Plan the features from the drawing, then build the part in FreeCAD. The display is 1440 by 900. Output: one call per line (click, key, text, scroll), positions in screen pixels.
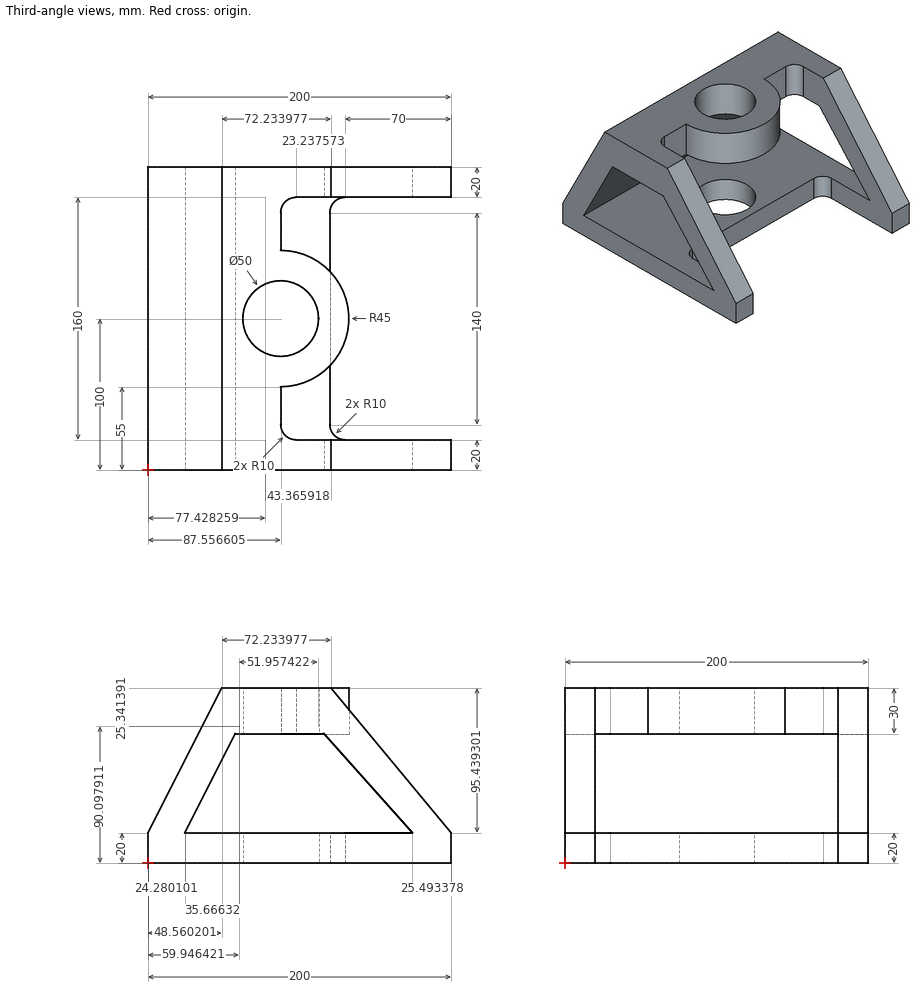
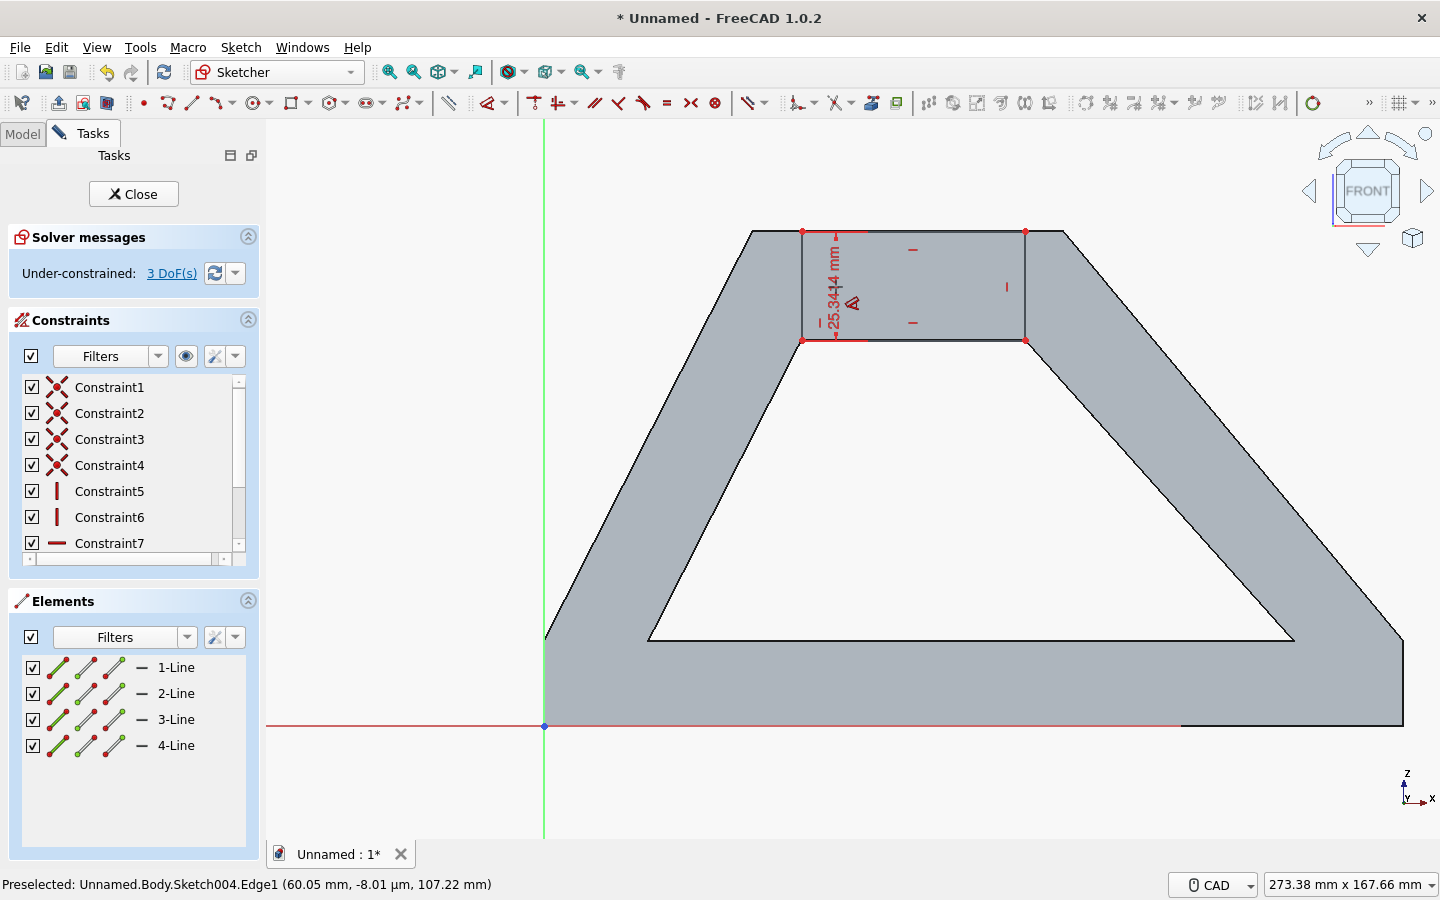
click(869, 341)
click(913, 307)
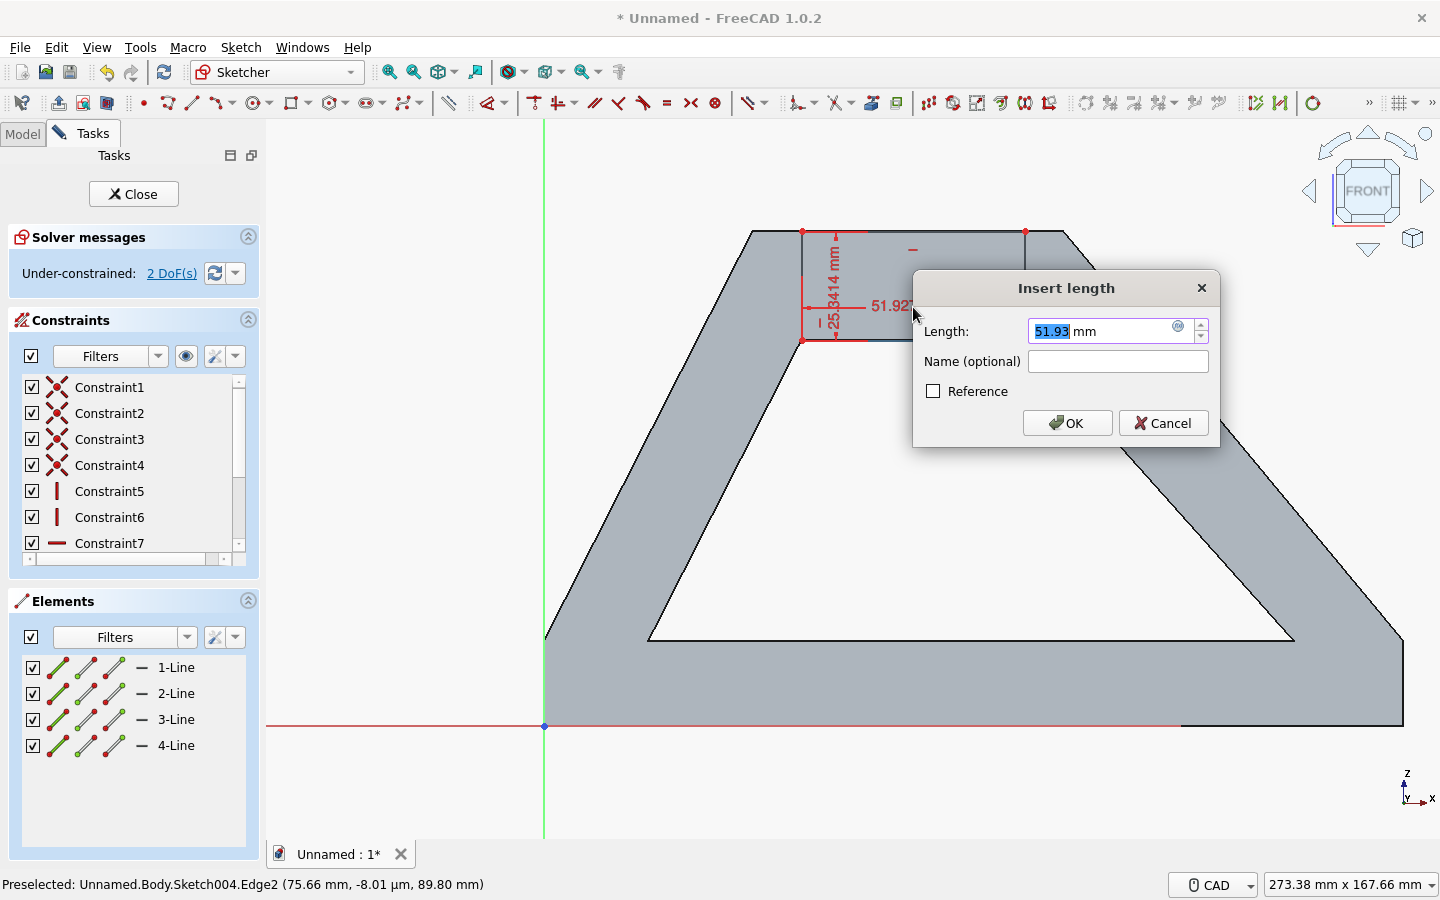
text(51.957422)
key(Return)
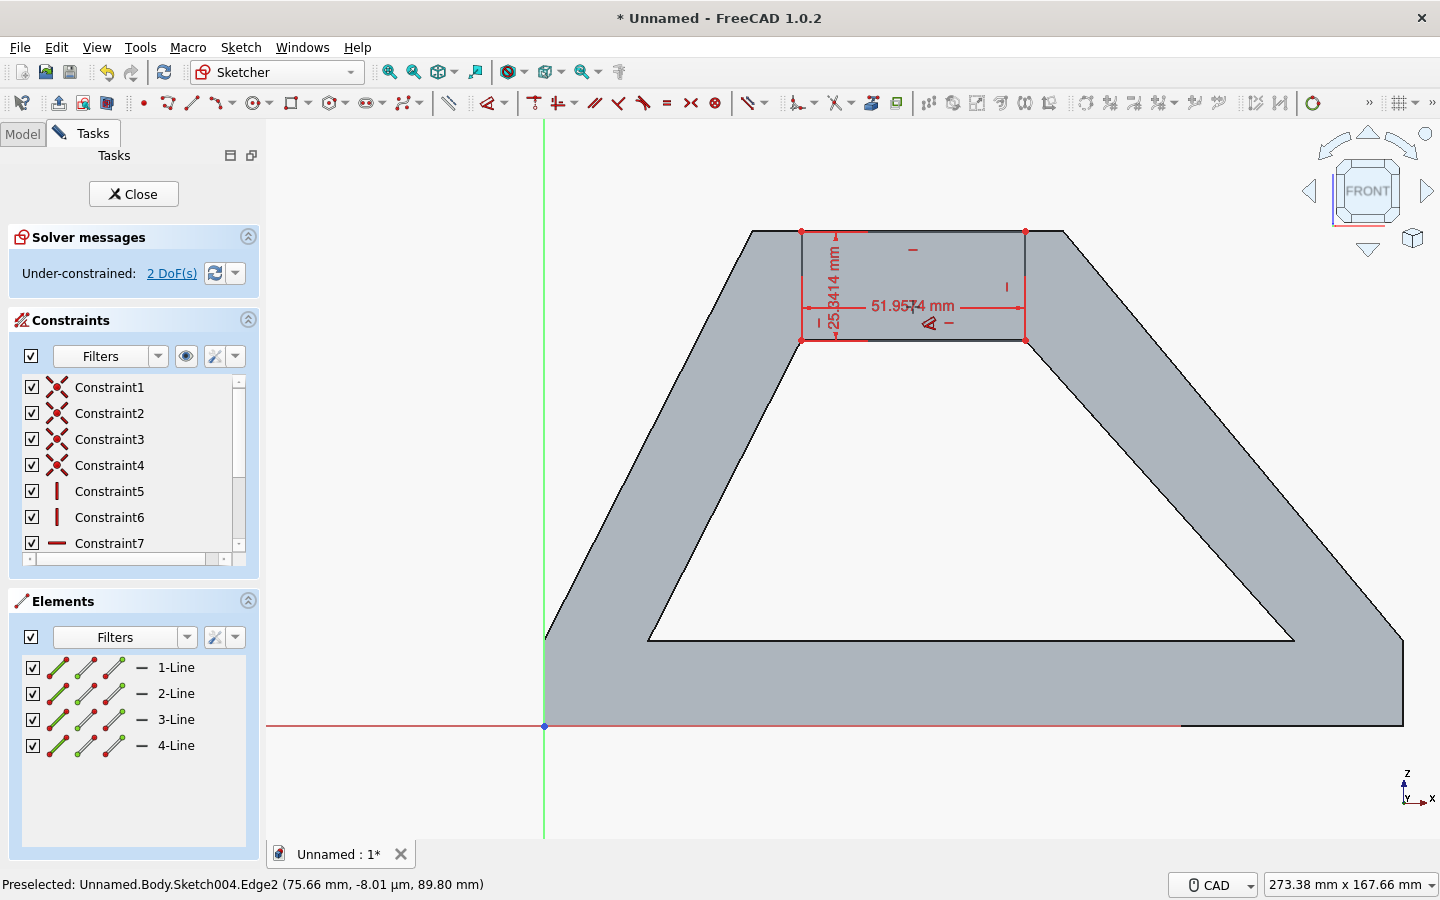
click(802, 232)
click(673, 760)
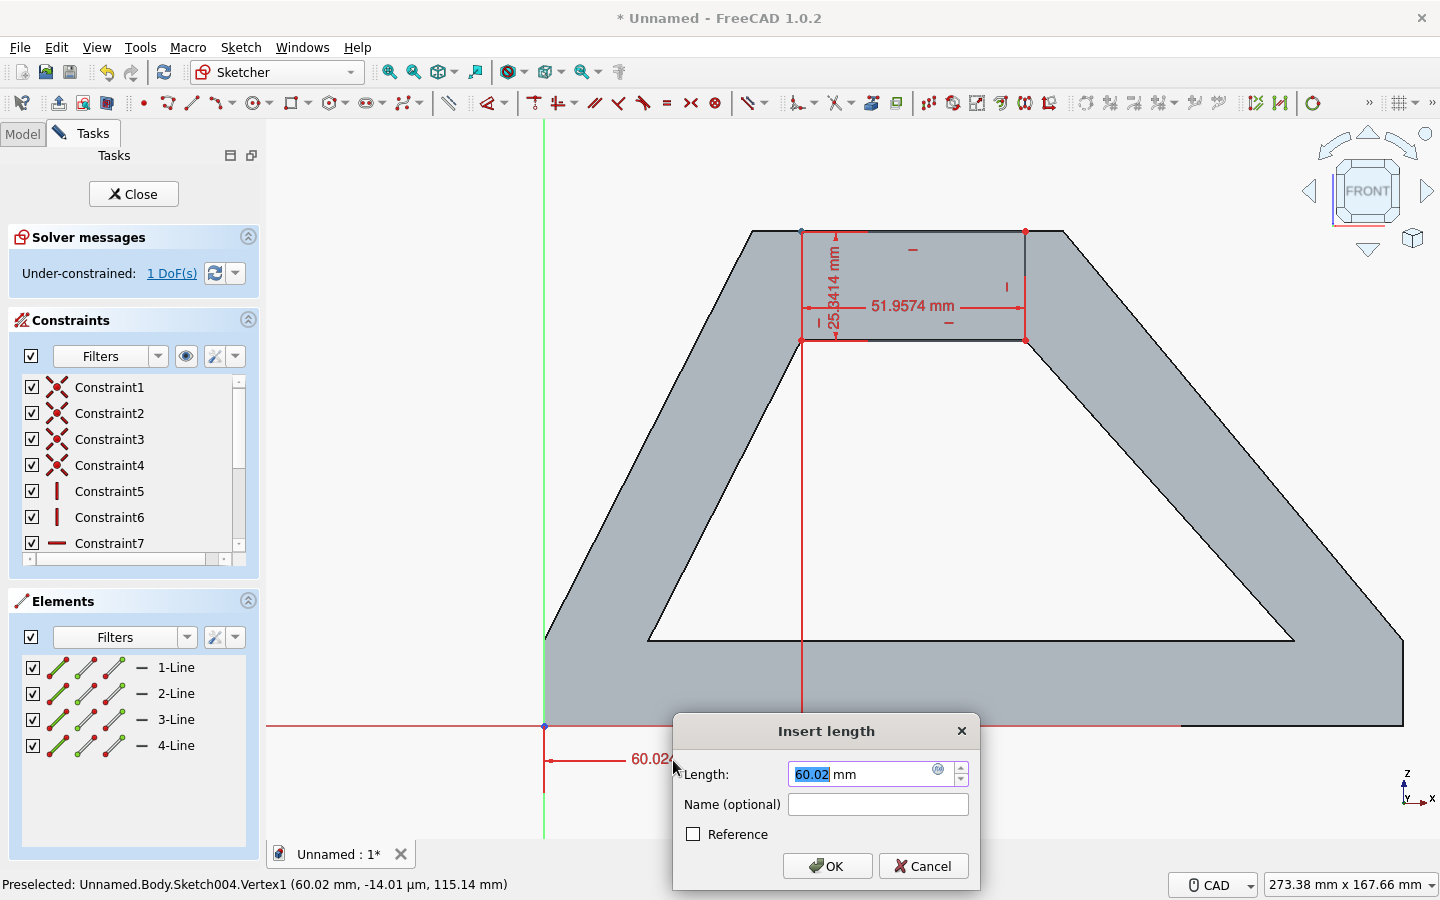
text(59.946421)
key(Return)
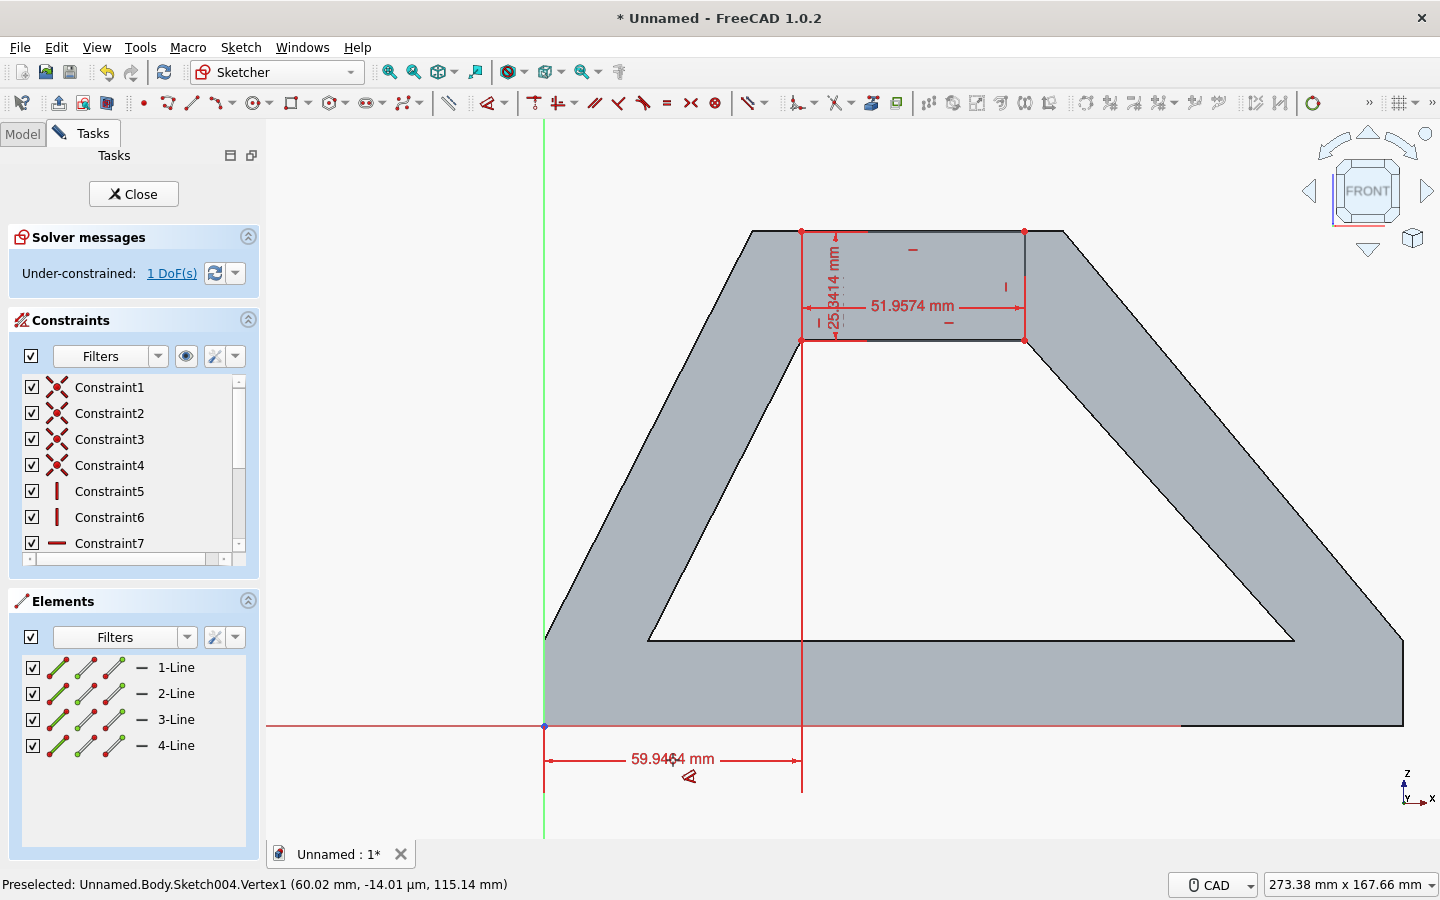
click(802, 341)
click(510, 534)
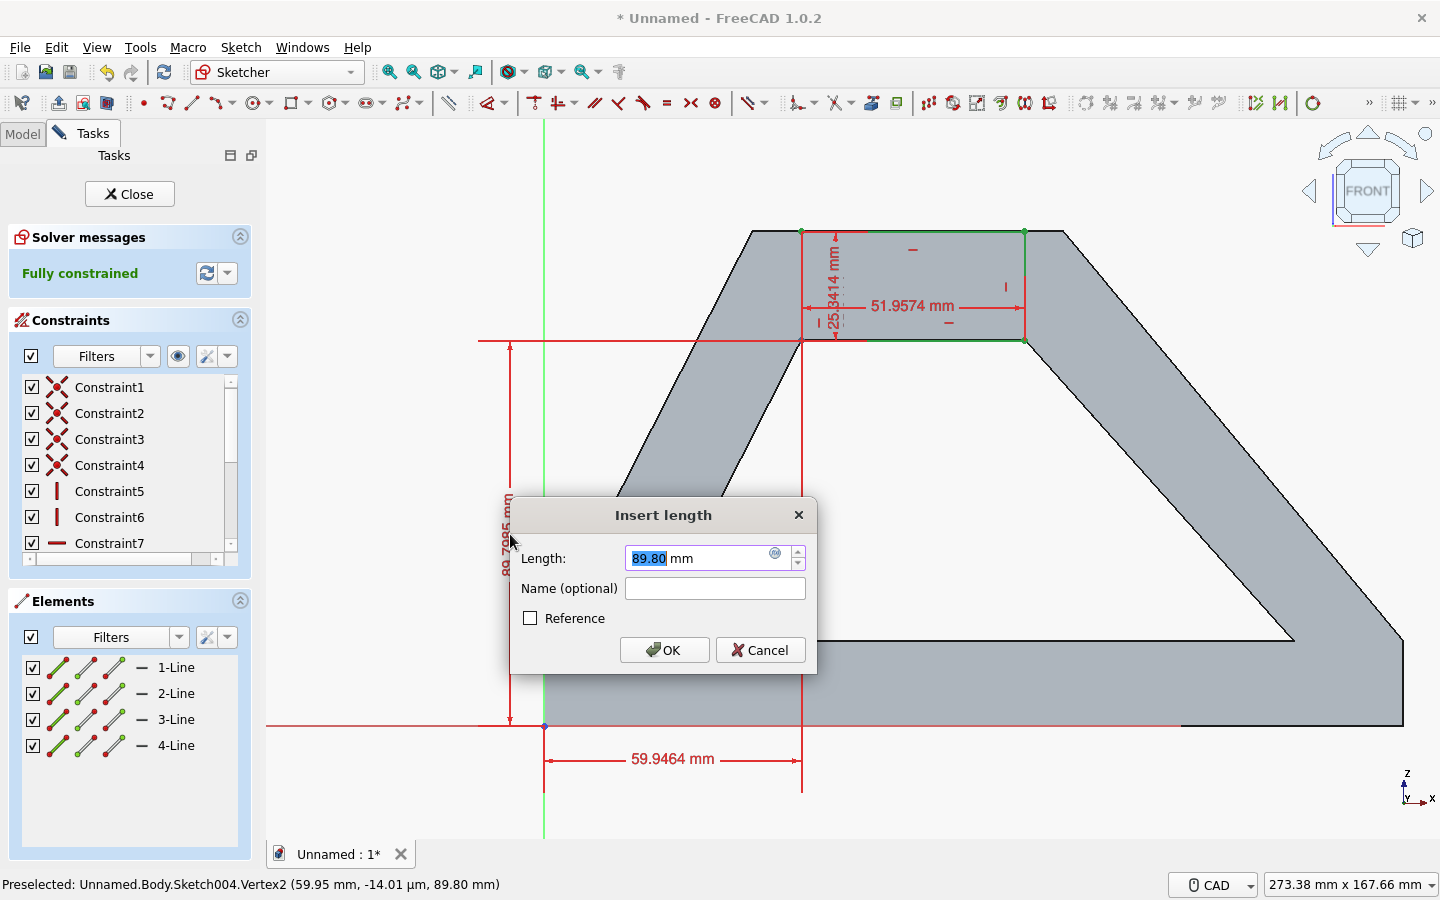
text(90.097911)
key(Return)
key(Escape)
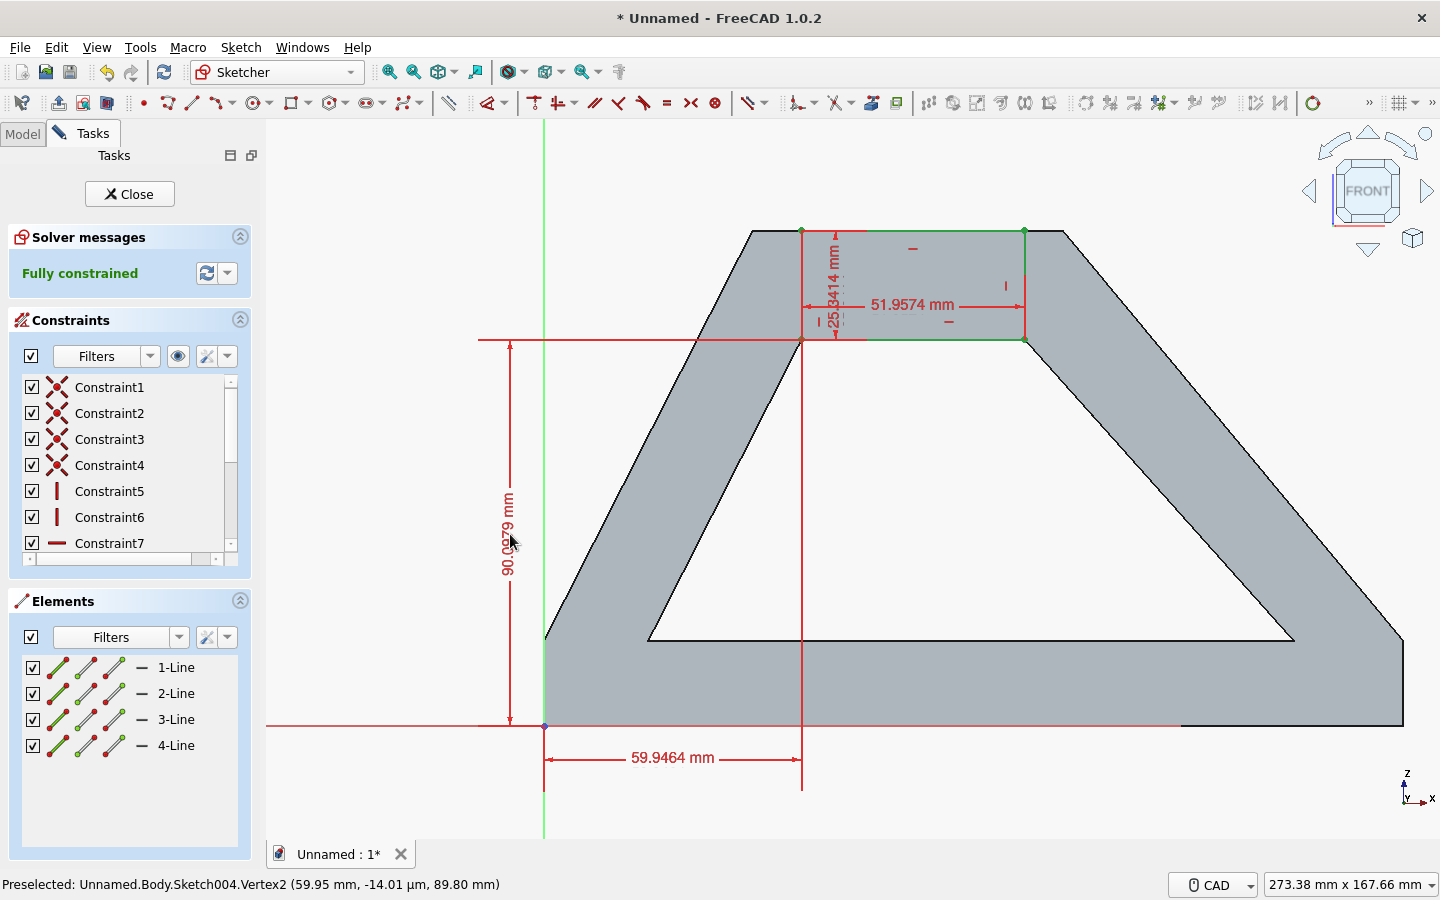
click(130, 194)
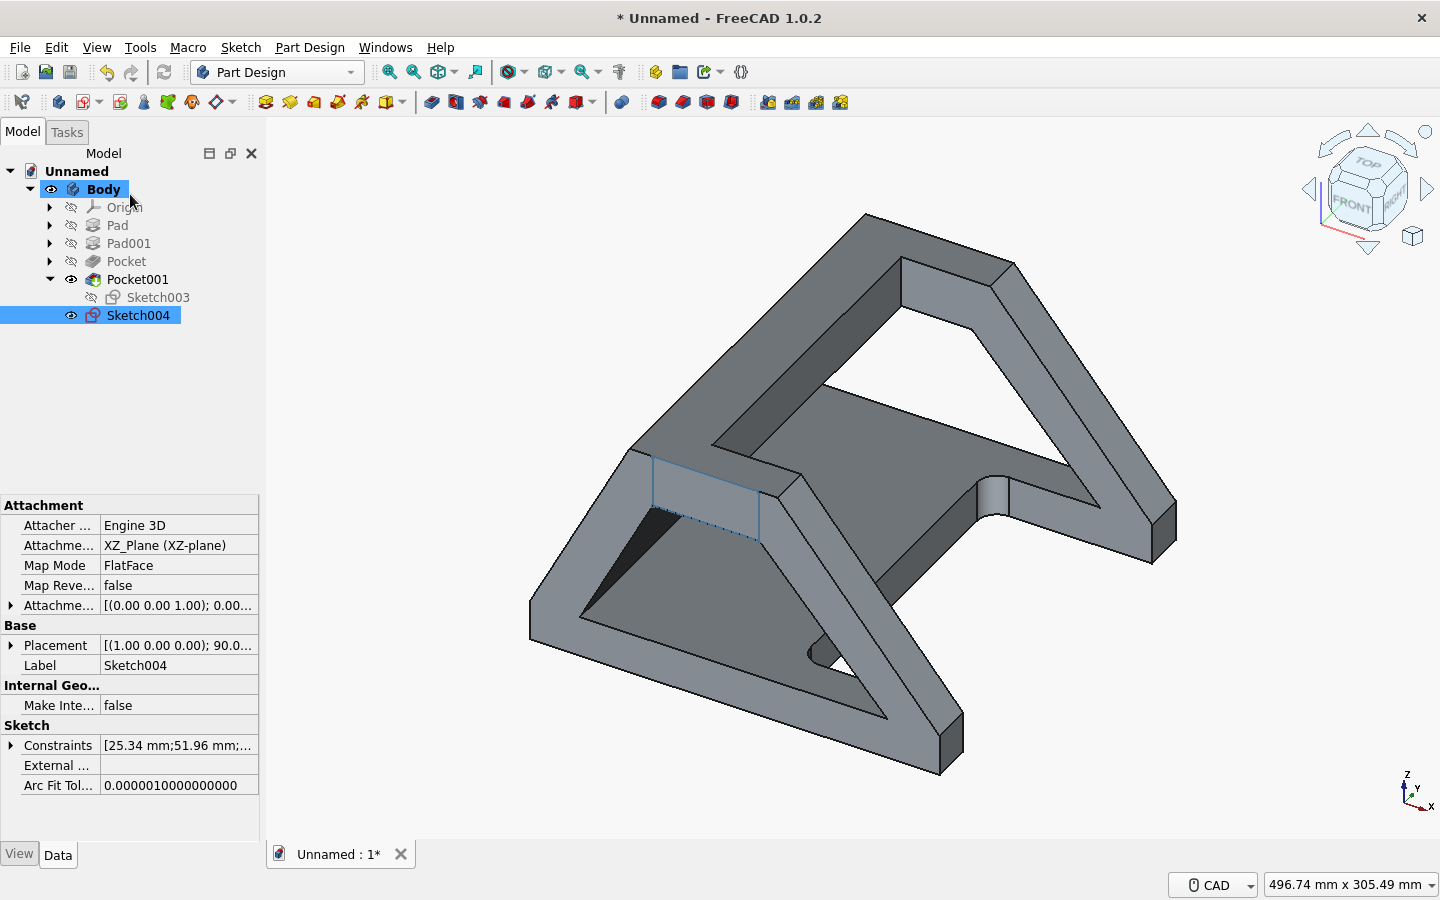
click(432, 102)